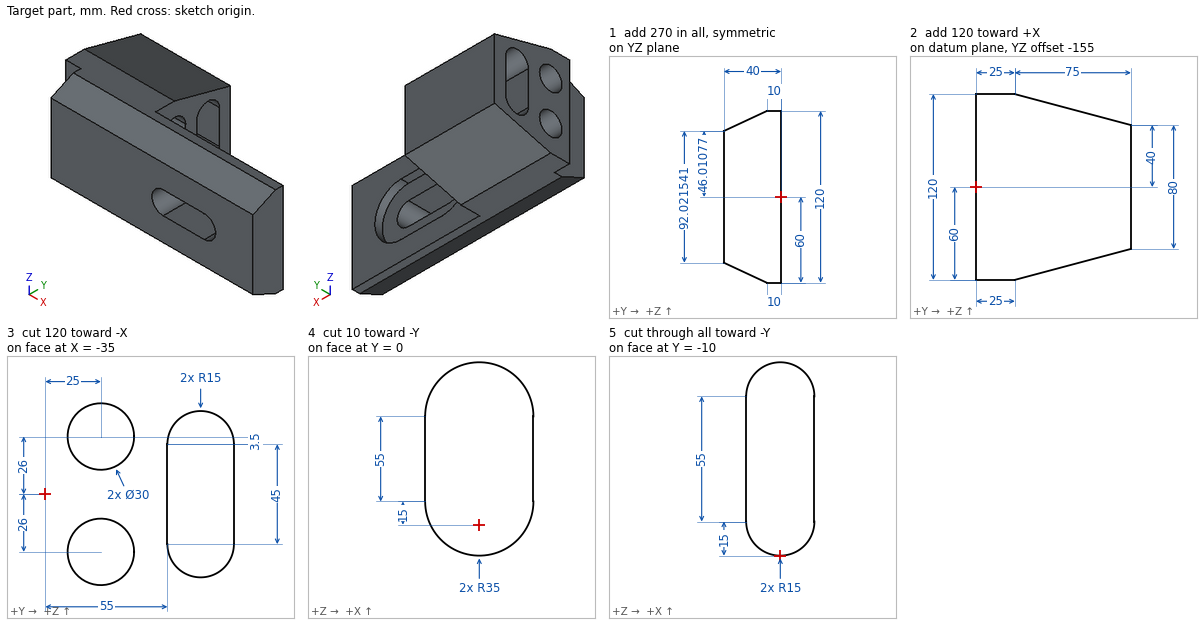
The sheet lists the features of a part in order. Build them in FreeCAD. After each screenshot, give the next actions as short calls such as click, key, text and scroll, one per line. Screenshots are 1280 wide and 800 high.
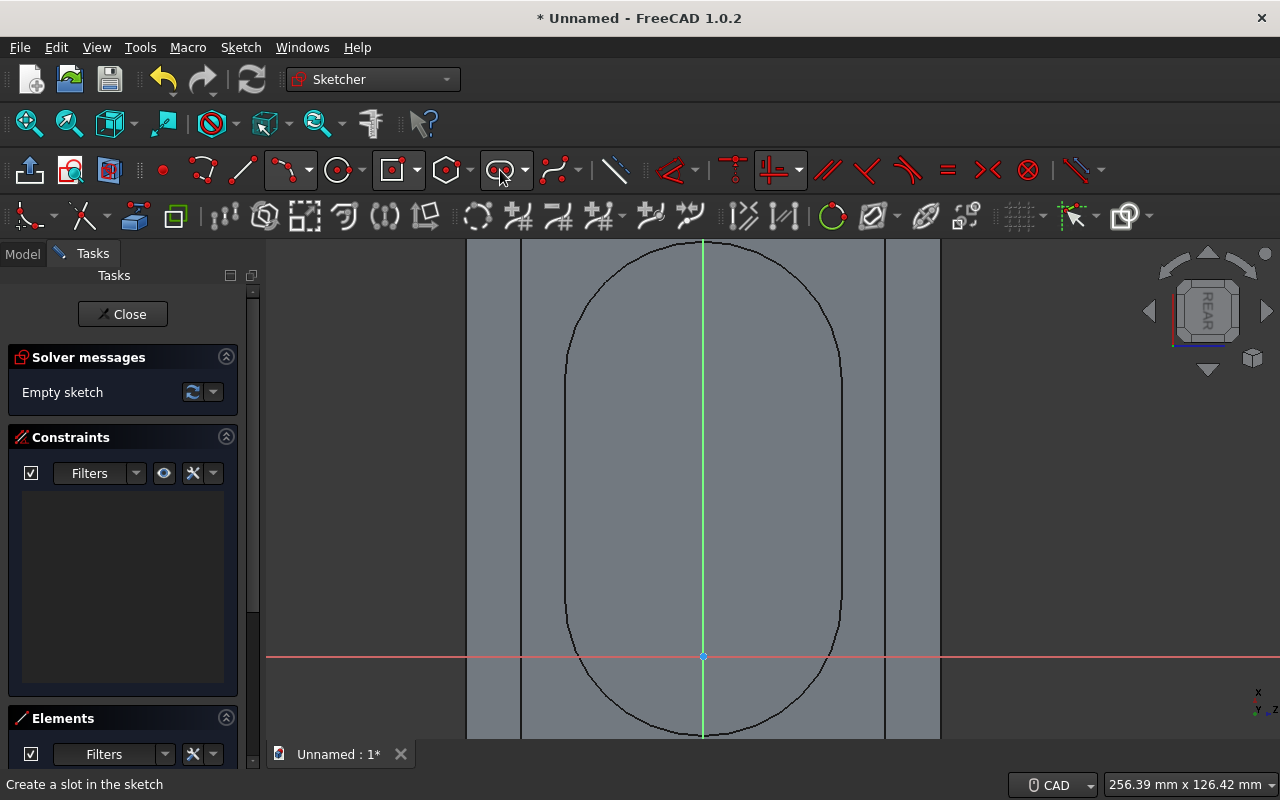
click(703, 598)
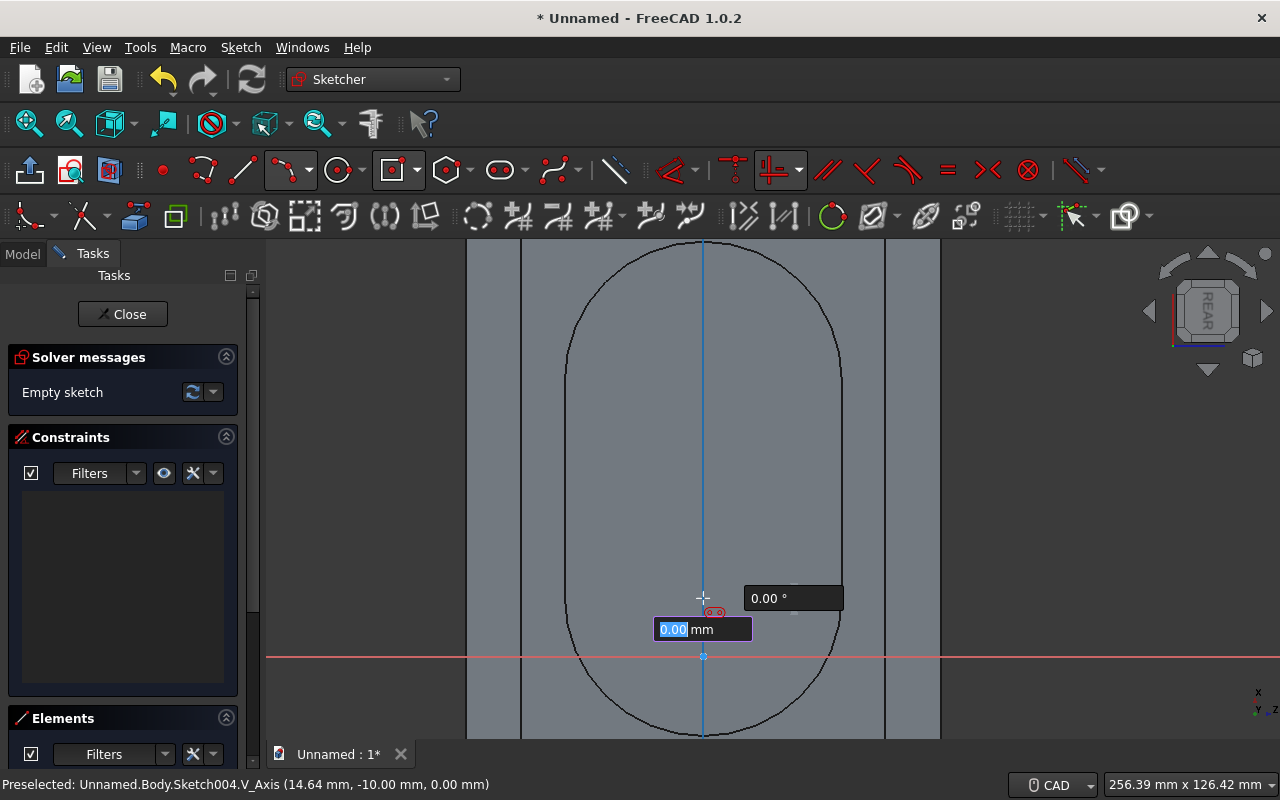
click(712, 380)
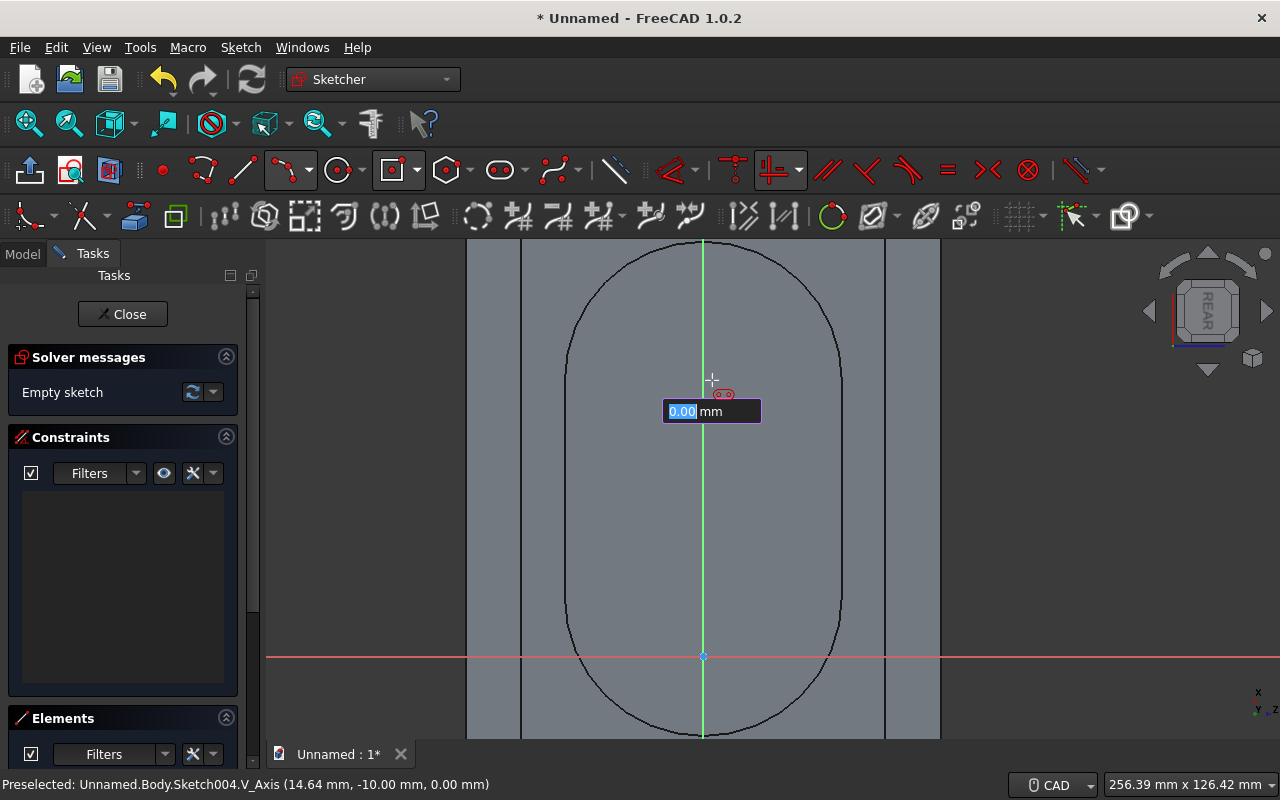
click(644, 489)
key(Escape)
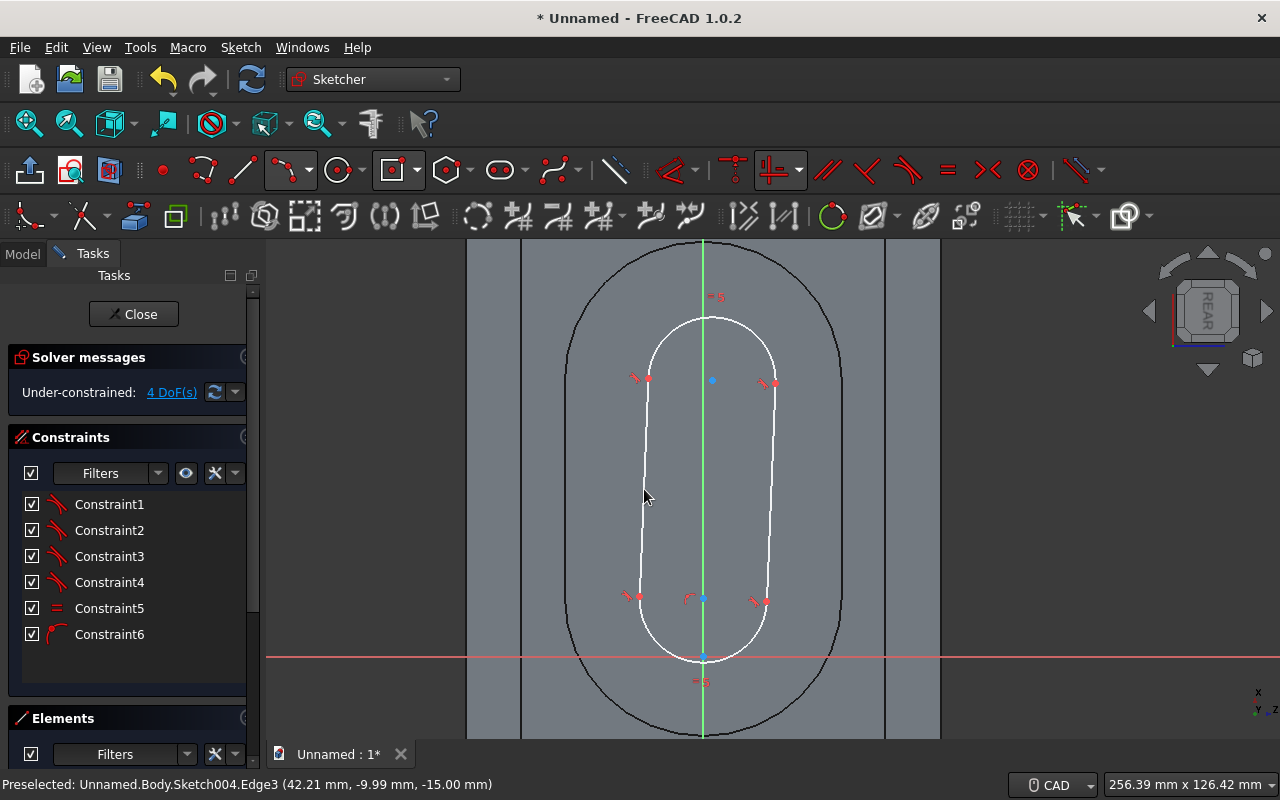
click(642, 531)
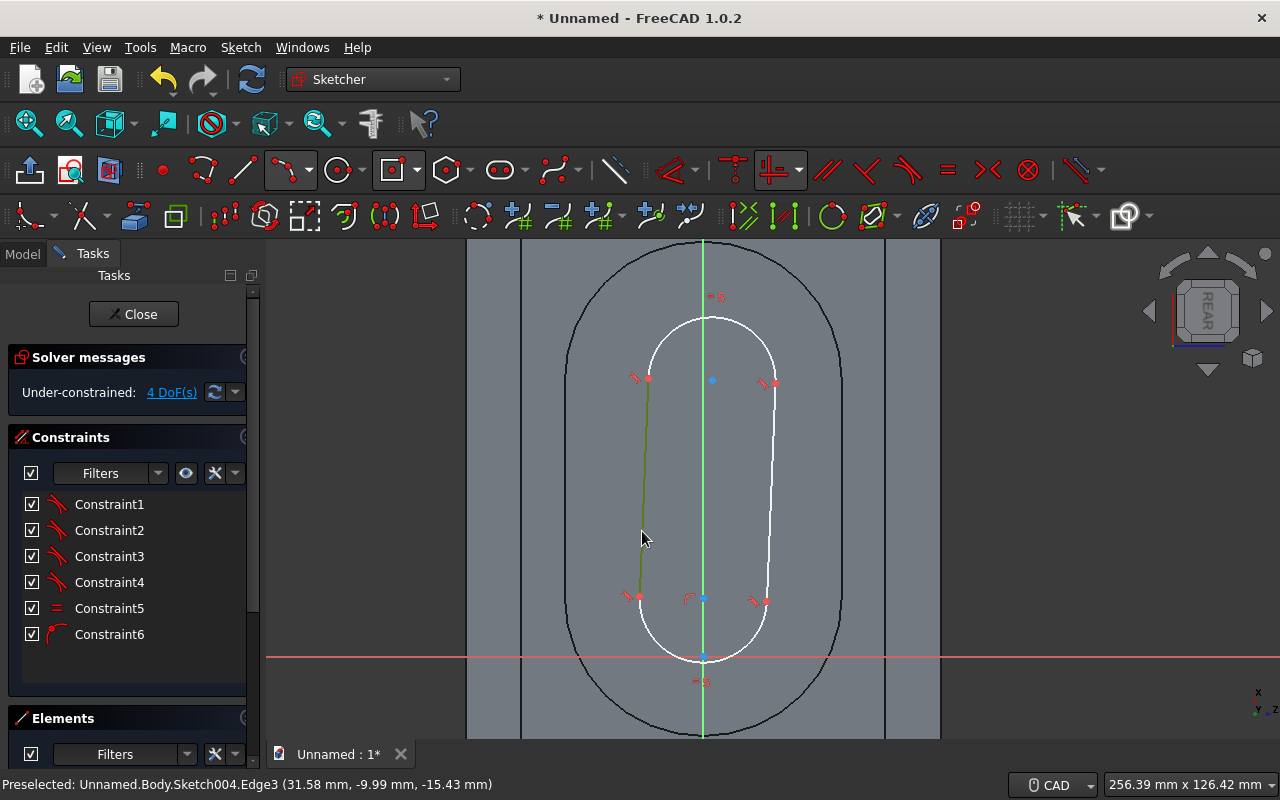
key(v)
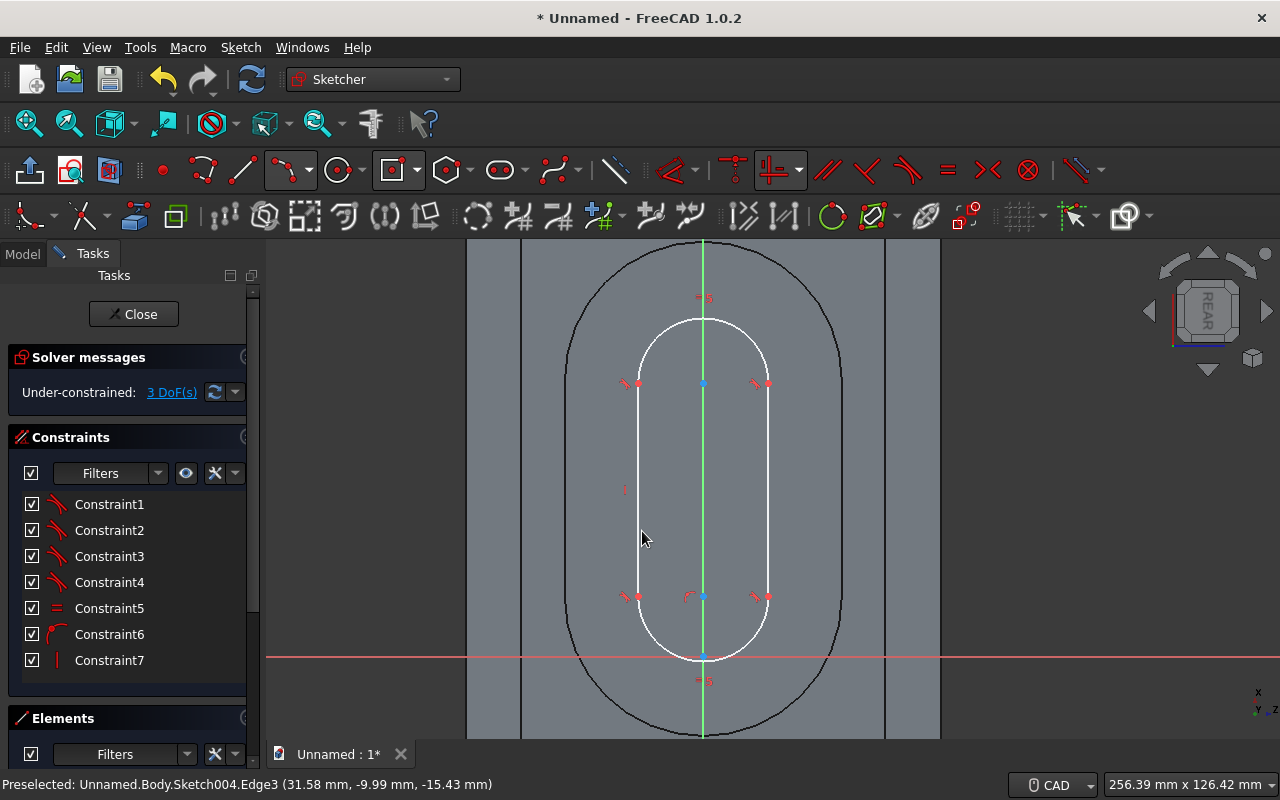
click(670, 170)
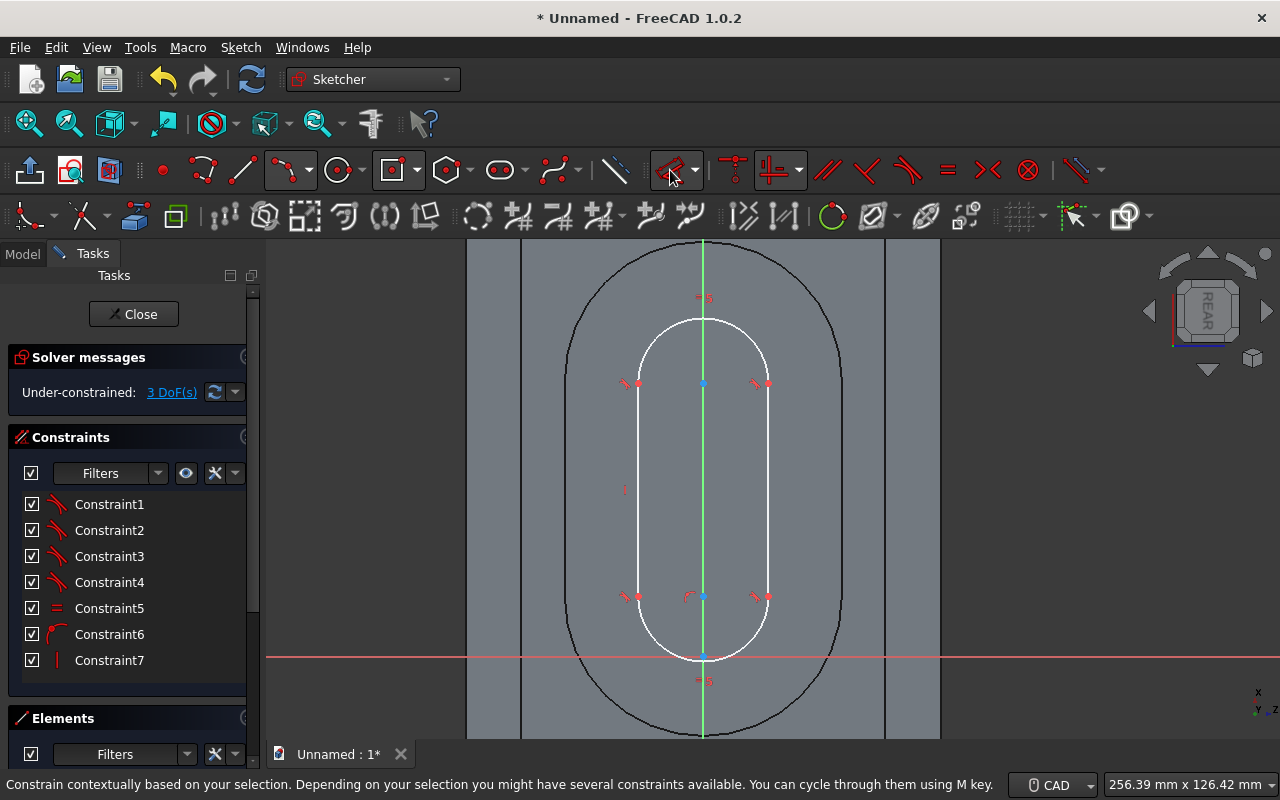
click(651, 635)
click(607, 609)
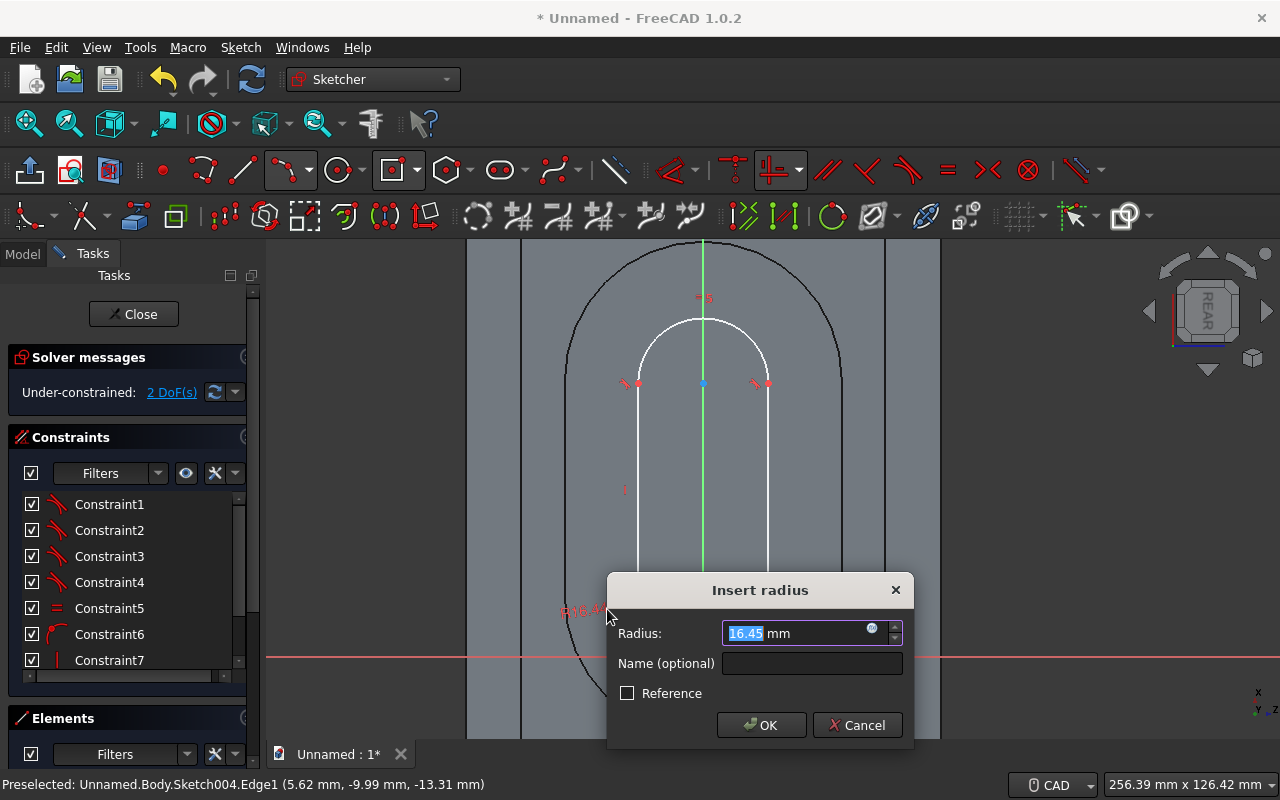
text(15)
key(Return)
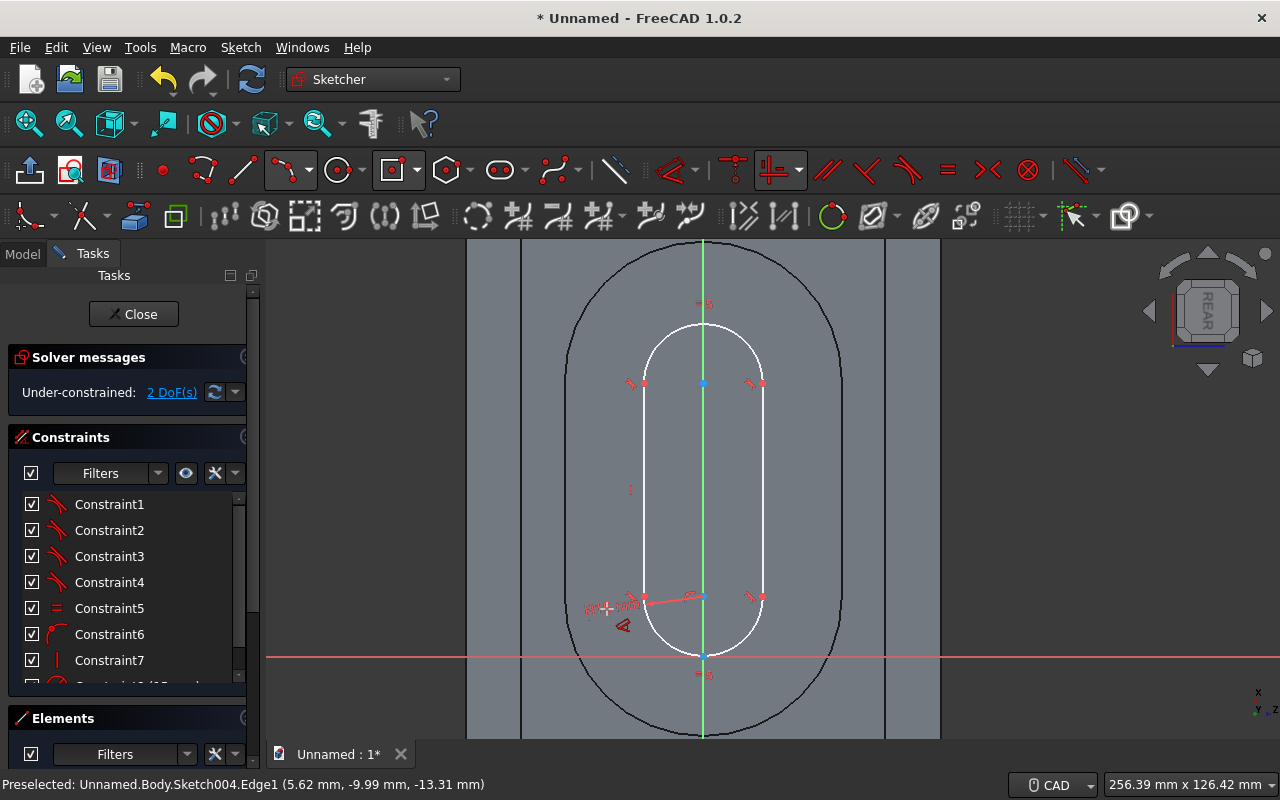
click(644, 533)
click(610, 490)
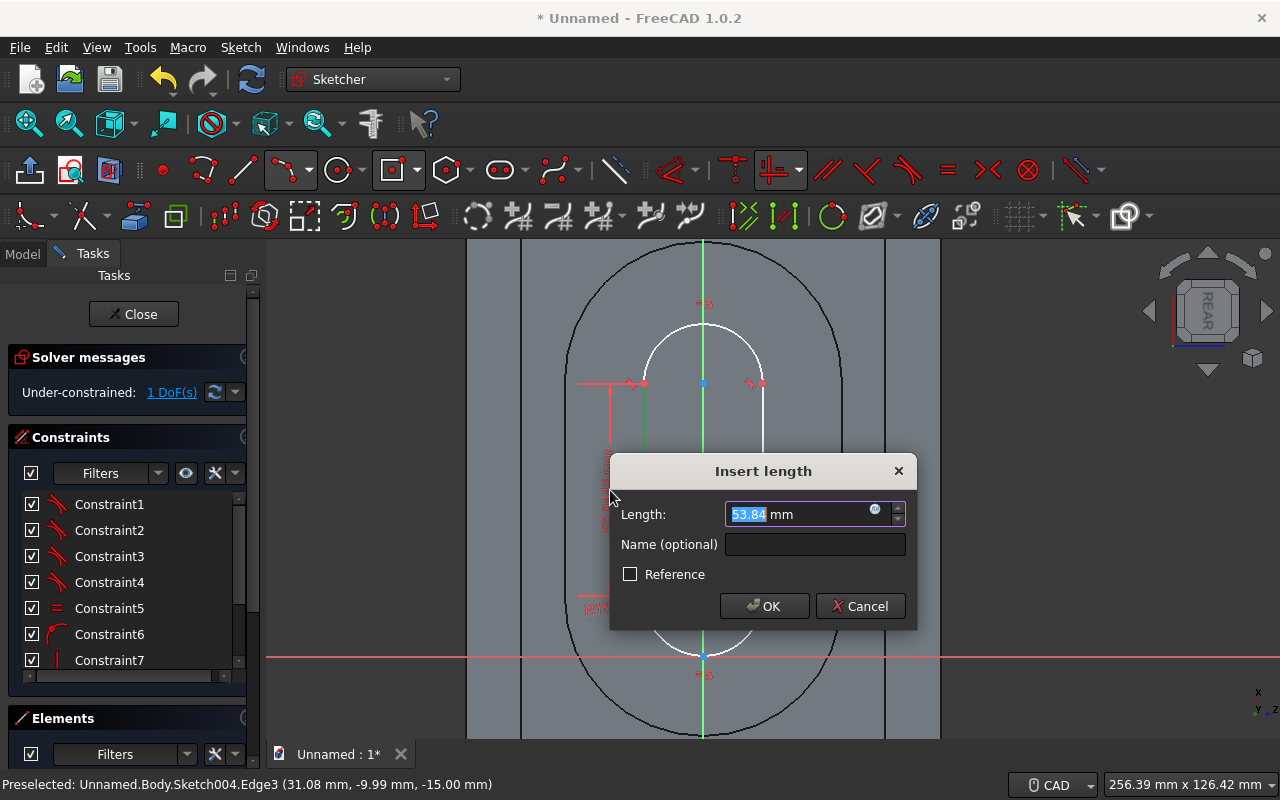
text(55)
key(Return)